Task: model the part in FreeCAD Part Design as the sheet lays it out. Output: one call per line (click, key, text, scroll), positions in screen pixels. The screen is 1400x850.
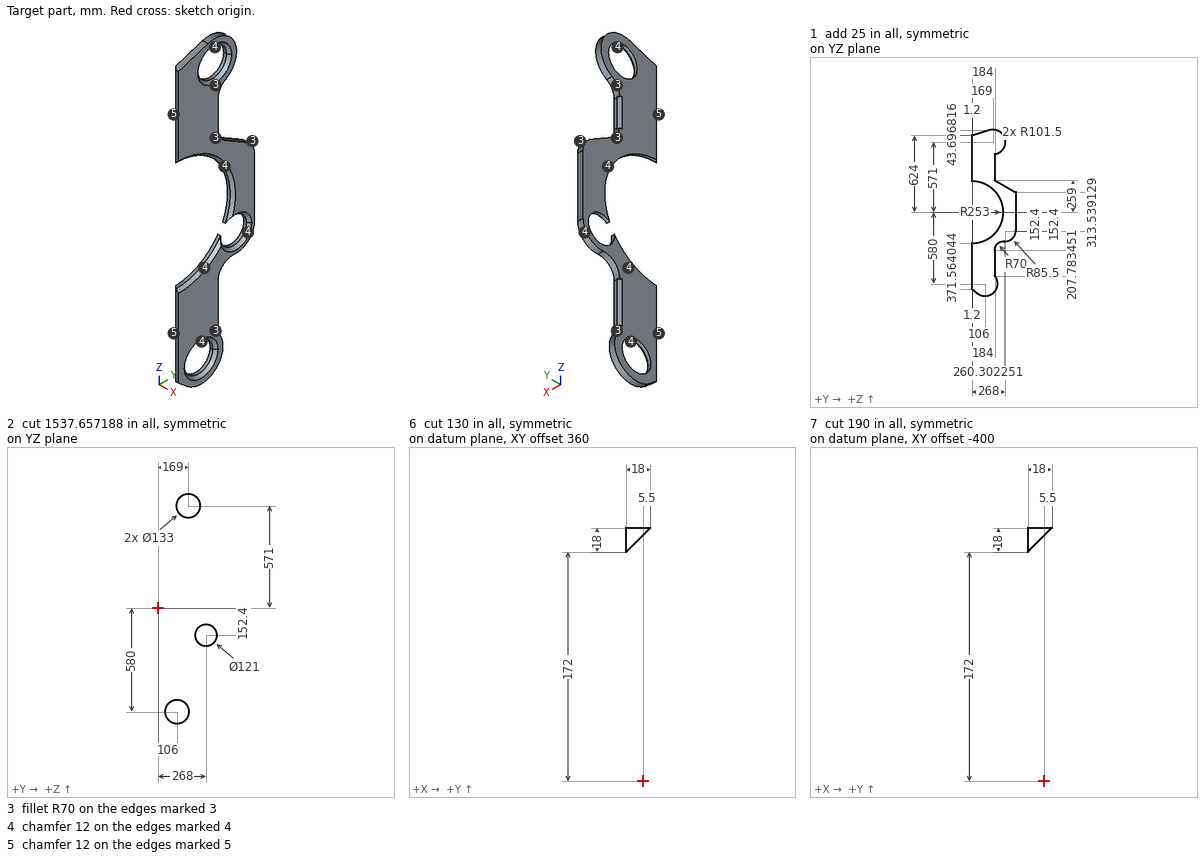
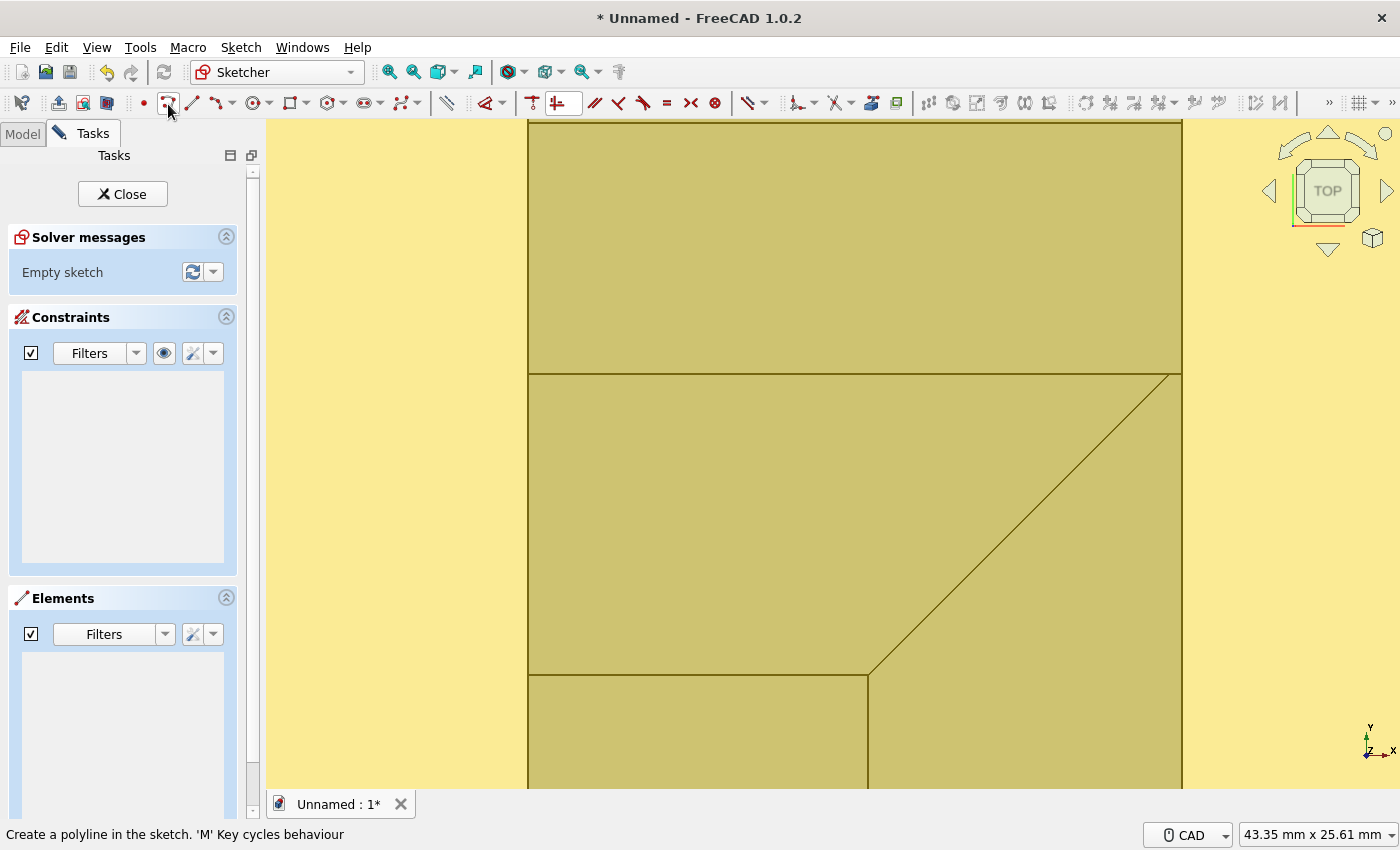
click(528, 688)
click(999, 217)
click(528, 217)
click(528, 689)
key(Escape)
key(Escape)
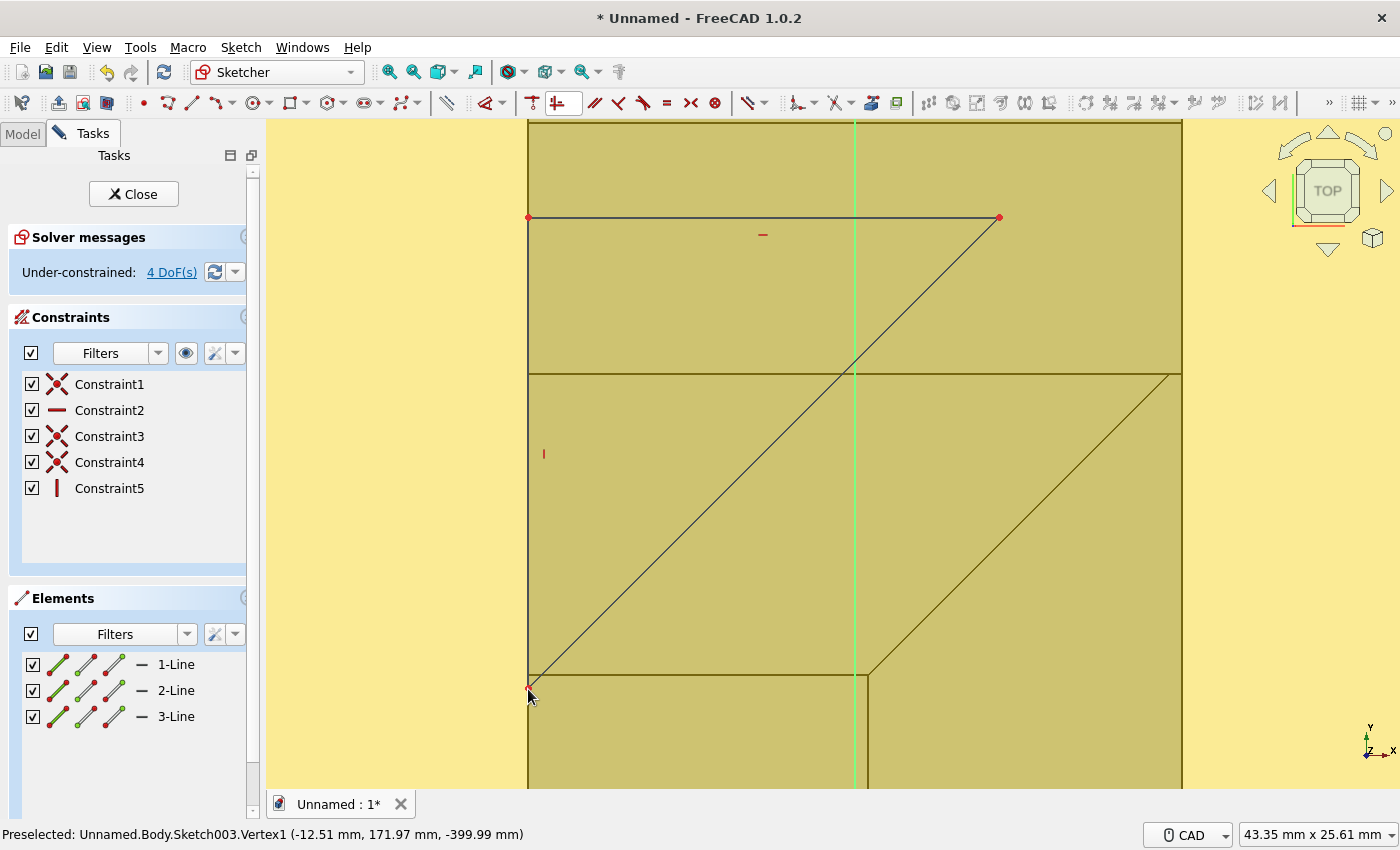
click(486, 104)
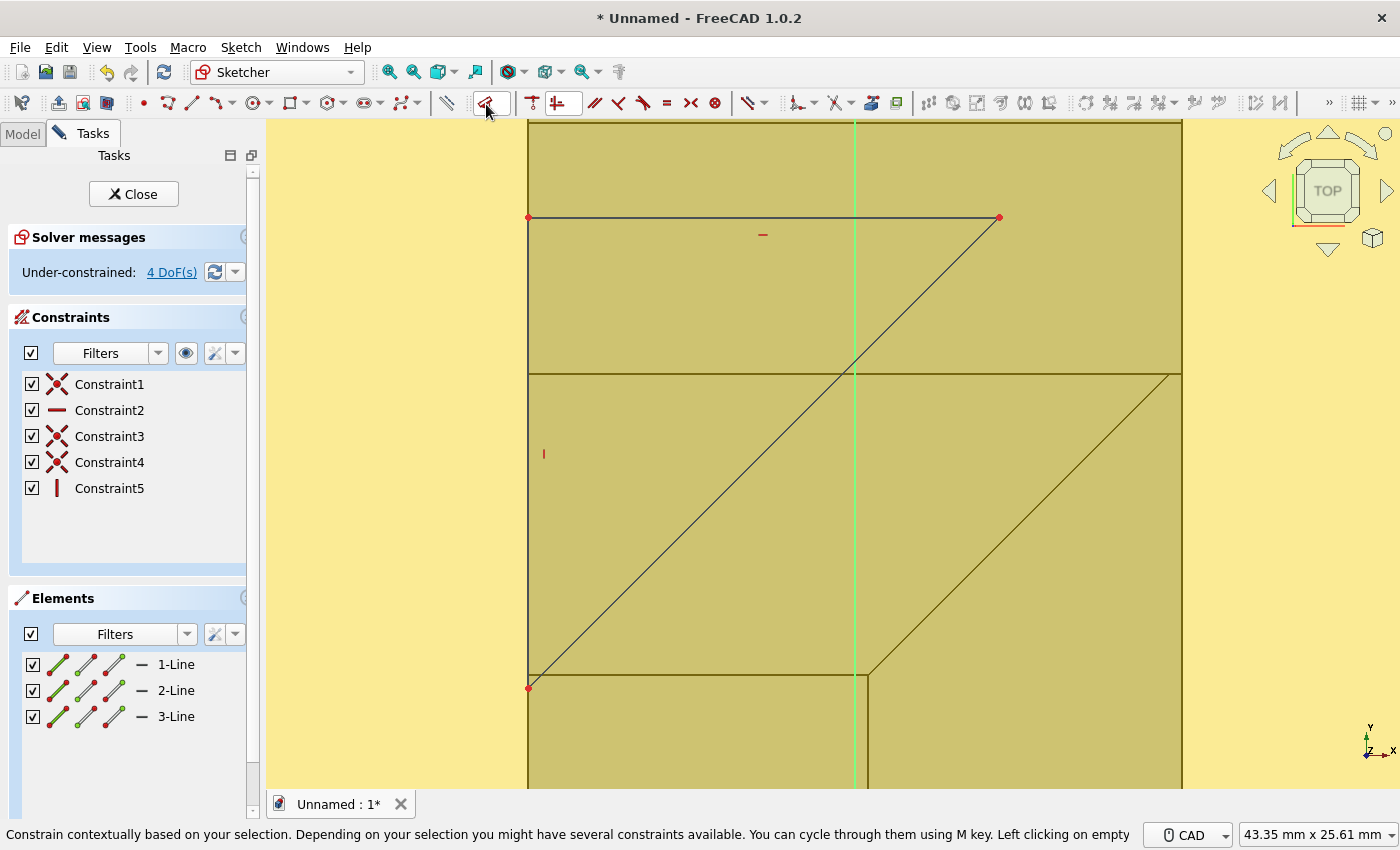
click(858, 218)
click(763, 184)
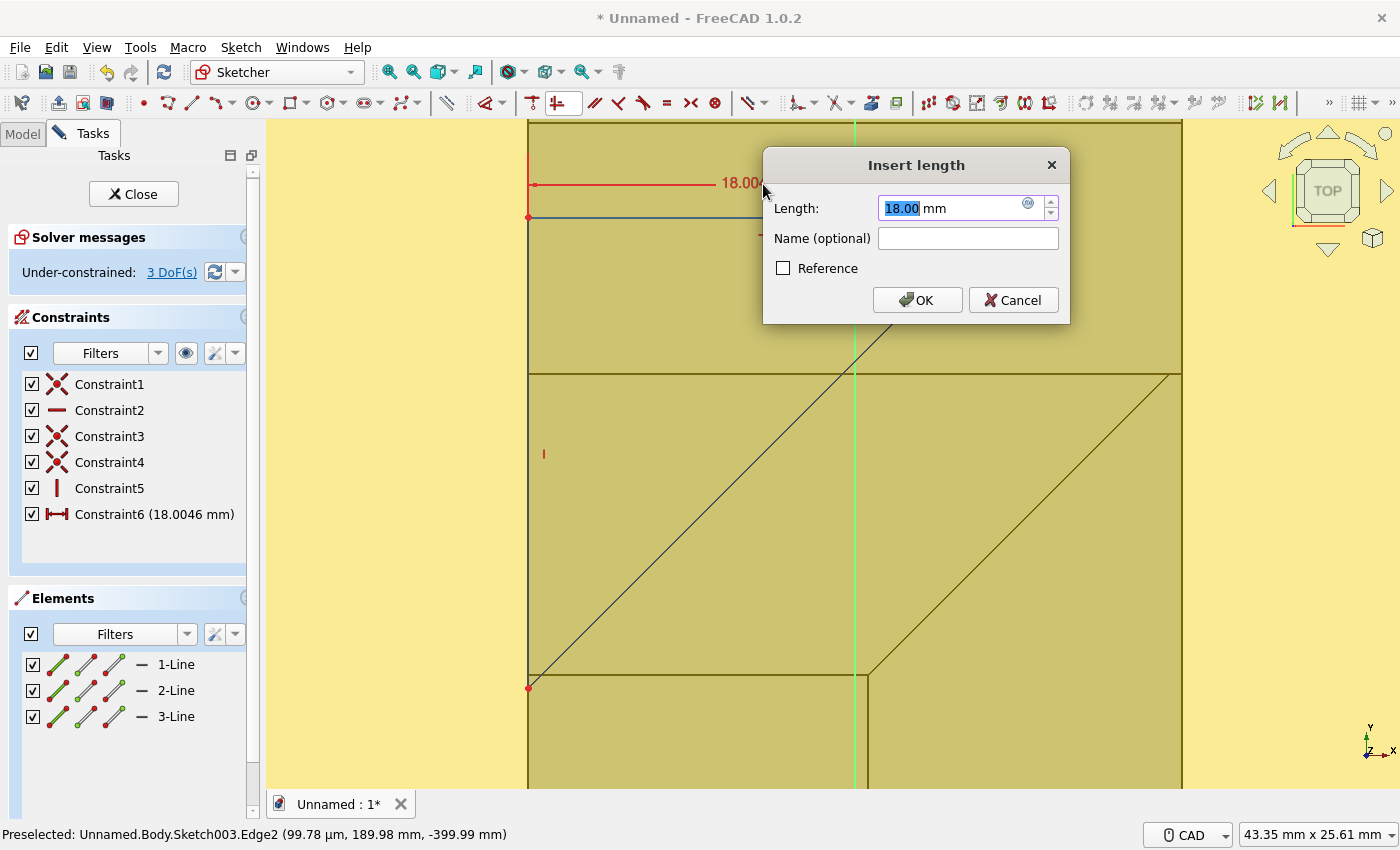
text(18)
key(Return)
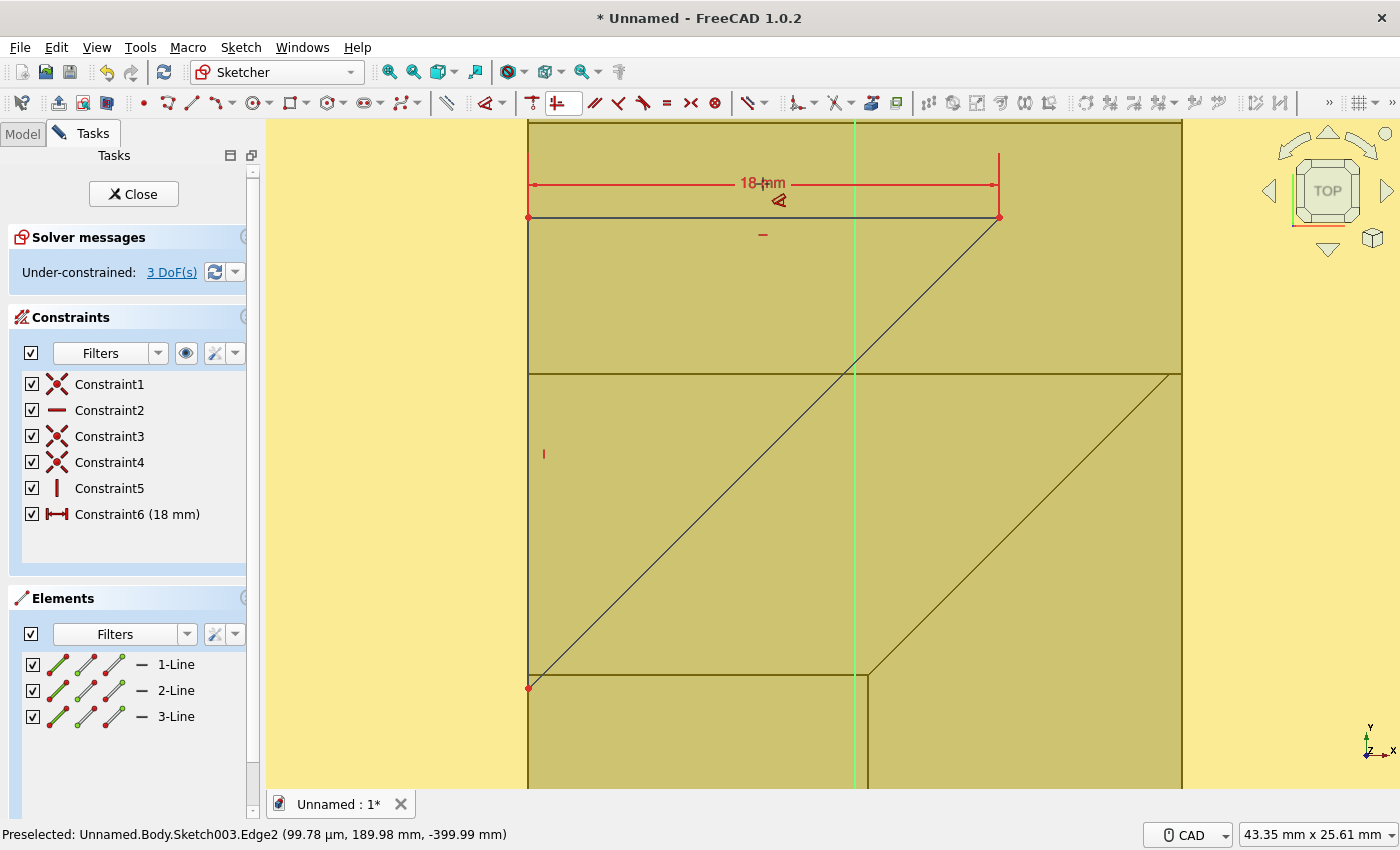
click(528, 359)
click(494, 454)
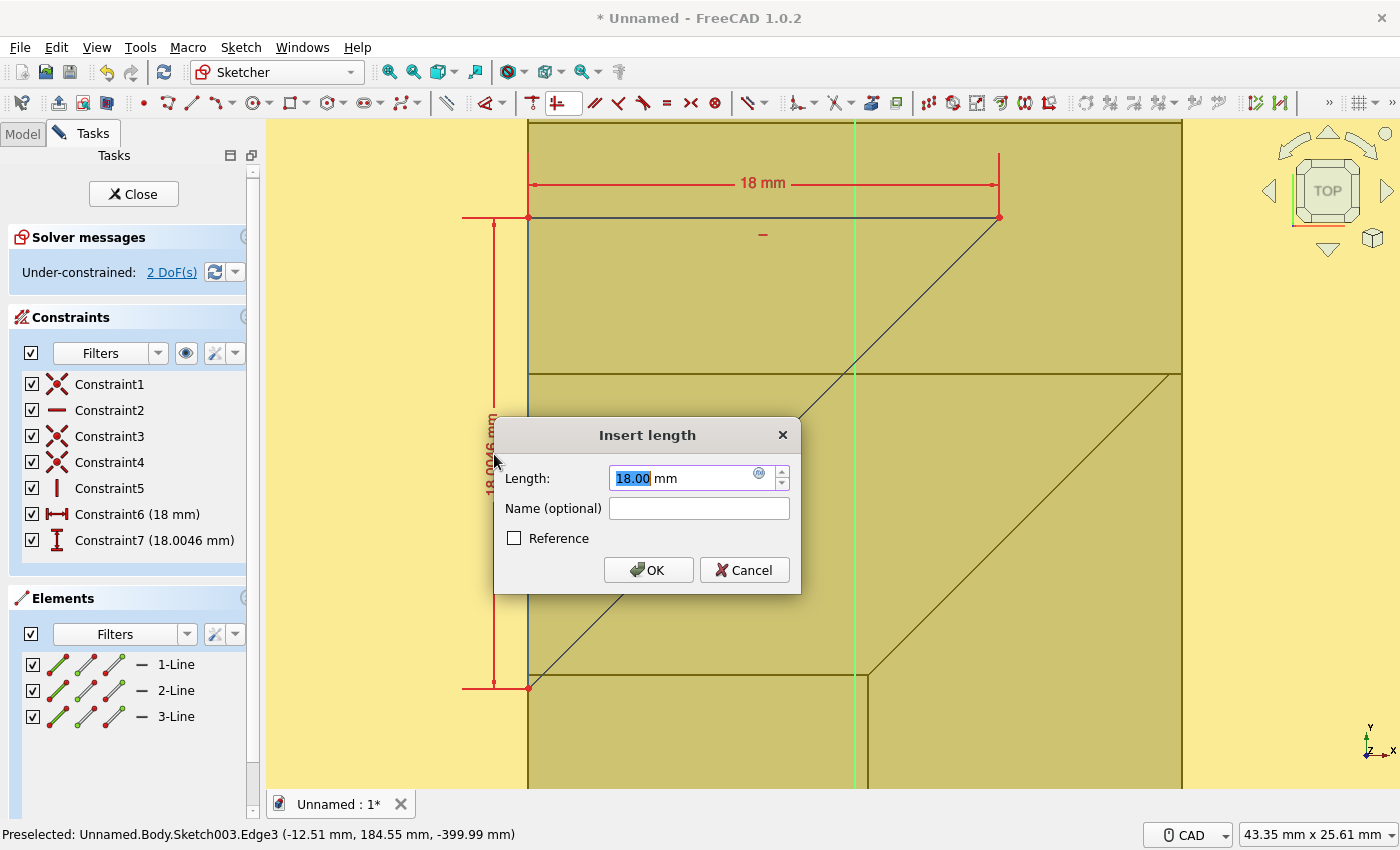
text(18)
key(Return)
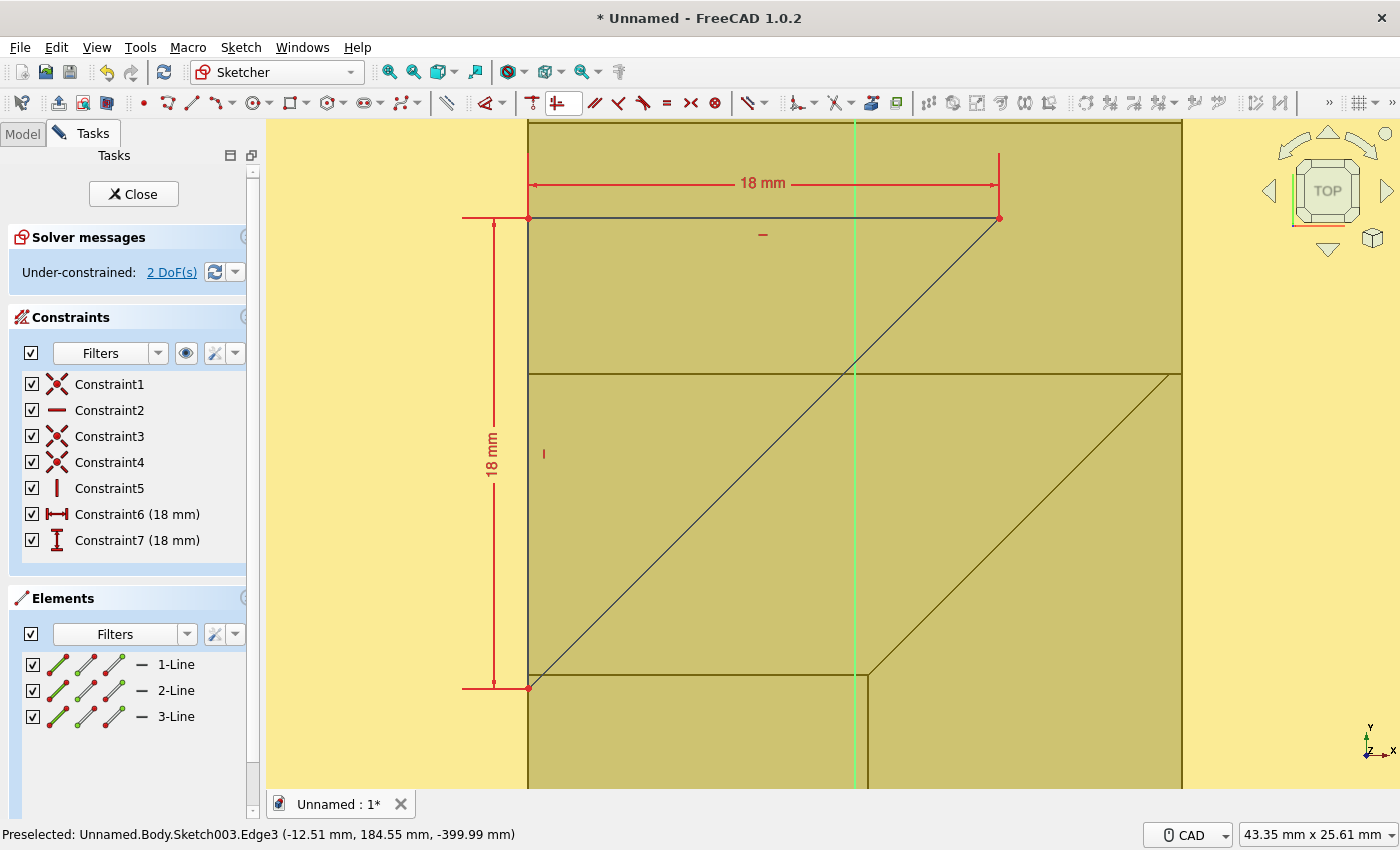
click(528, 689)
click(494, 725)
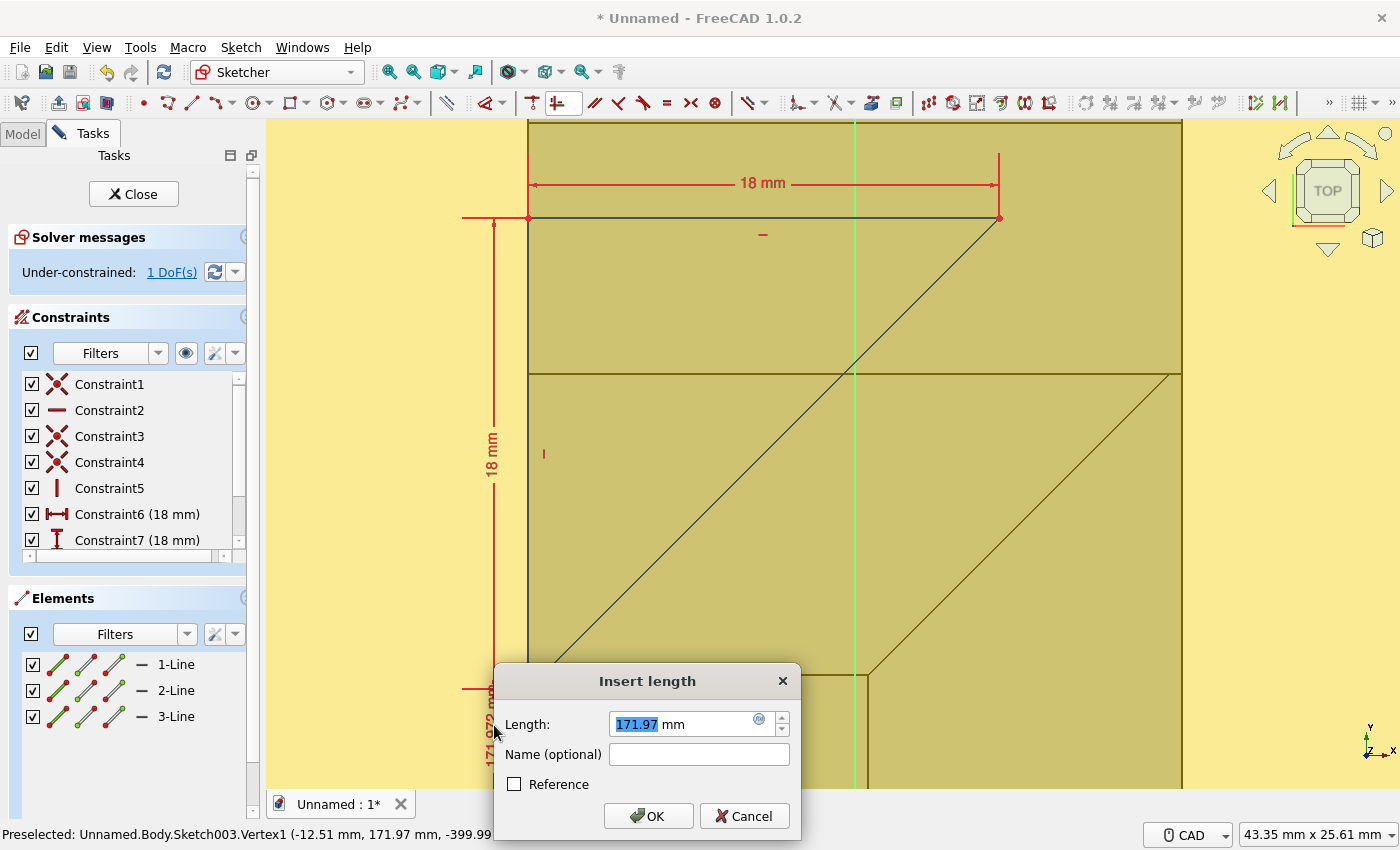
text(172)
key(Return)